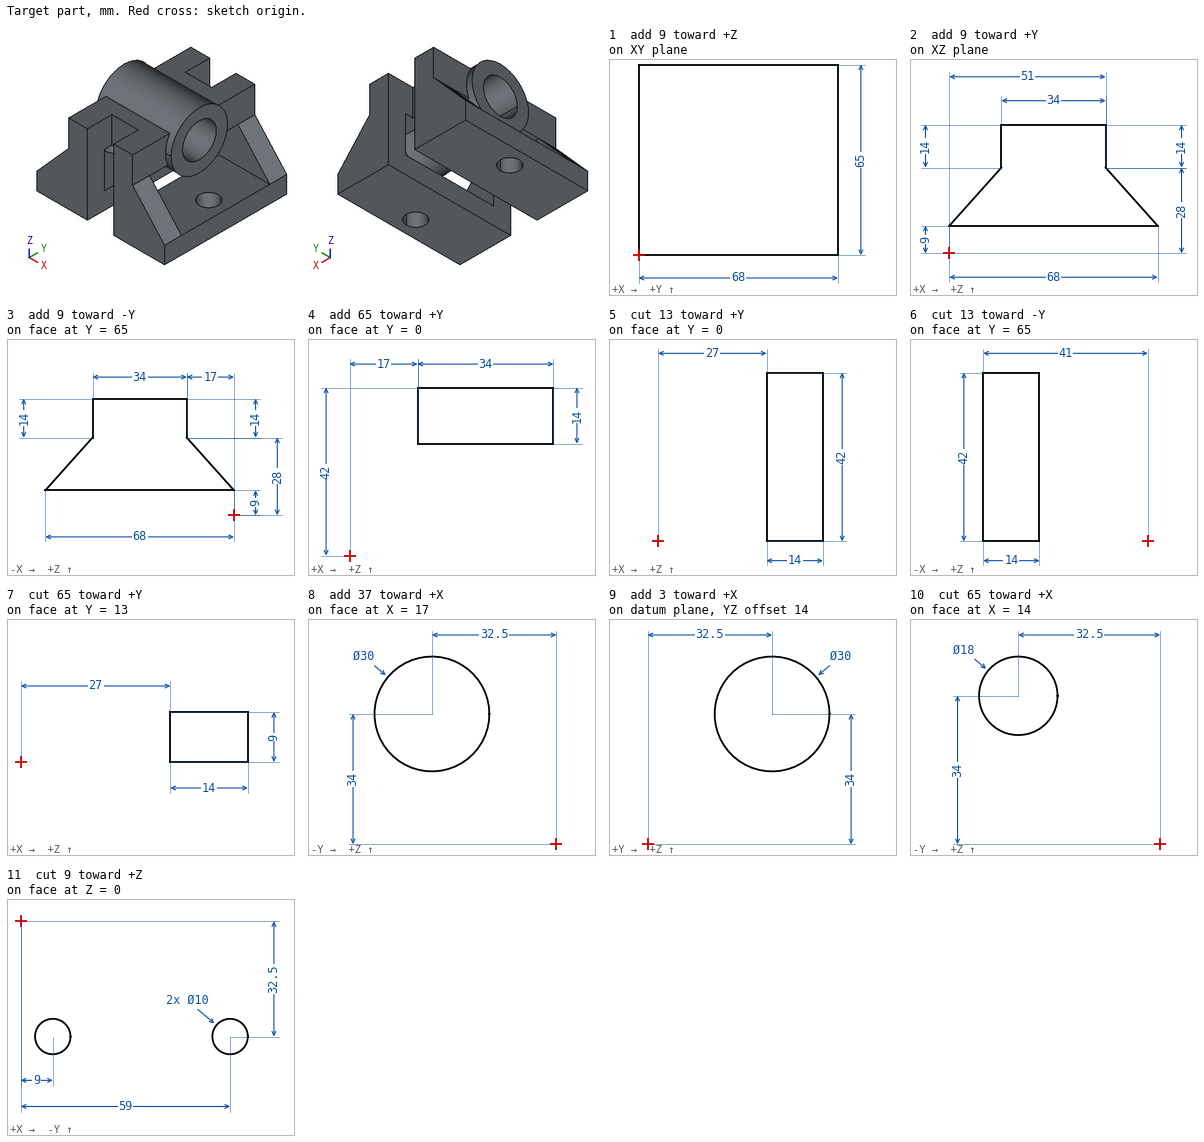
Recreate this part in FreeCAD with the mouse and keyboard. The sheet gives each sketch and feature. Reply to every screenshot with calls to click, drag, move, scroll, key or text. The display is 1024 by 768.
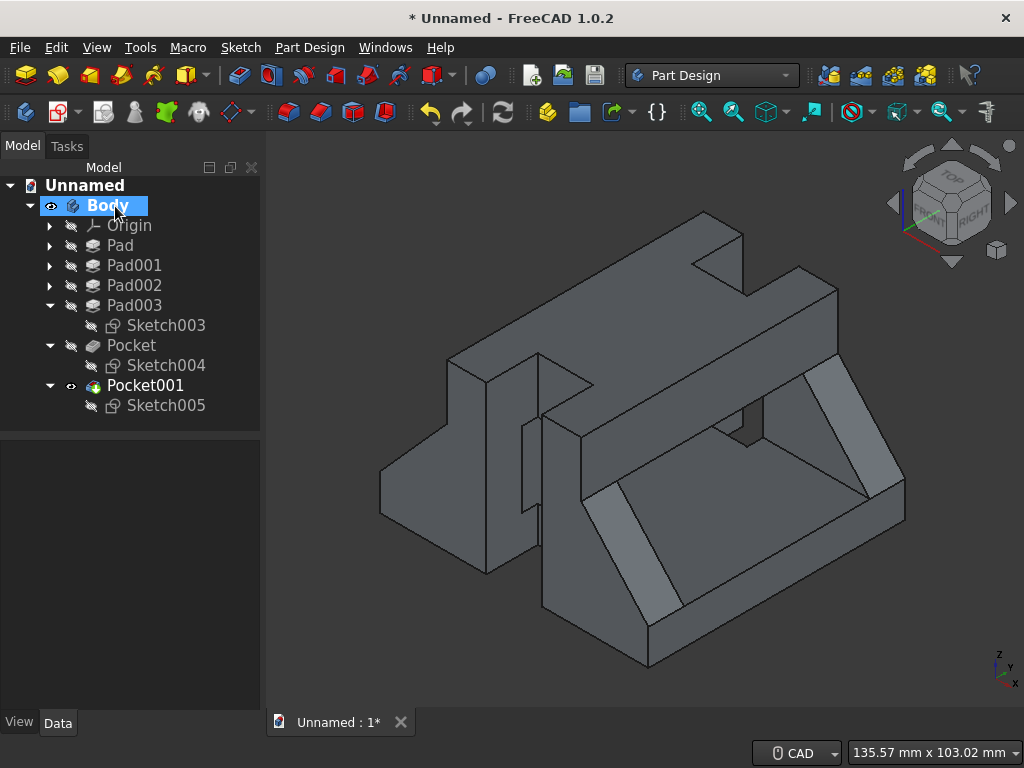
click(558, 386)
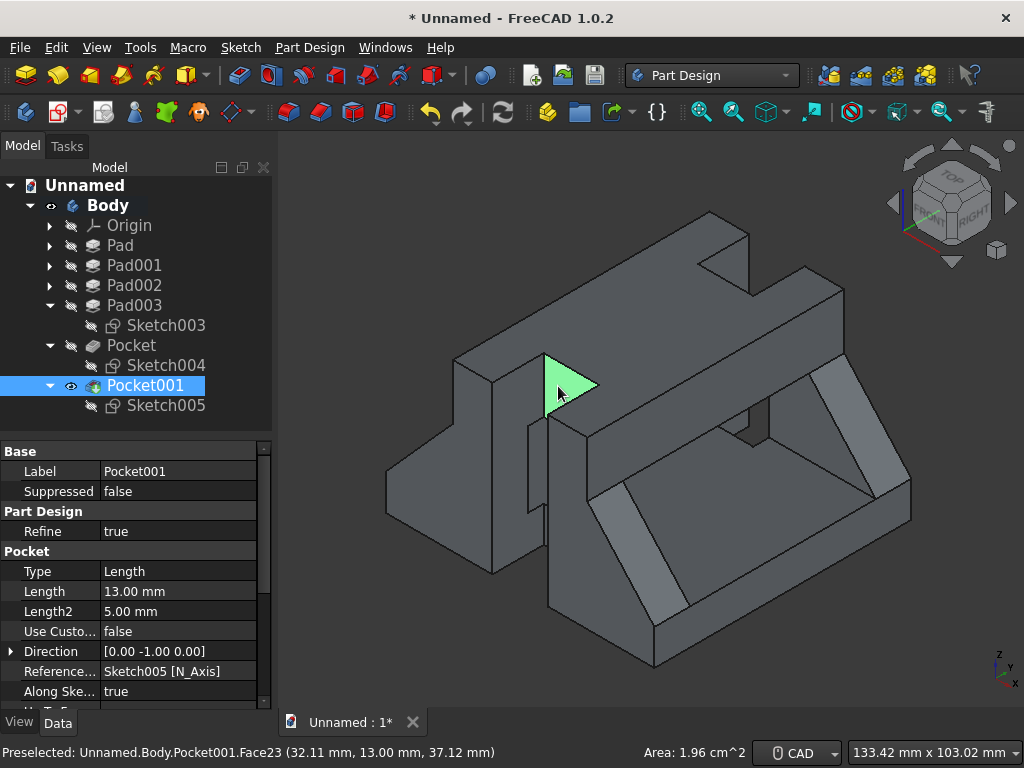
click(58, 112)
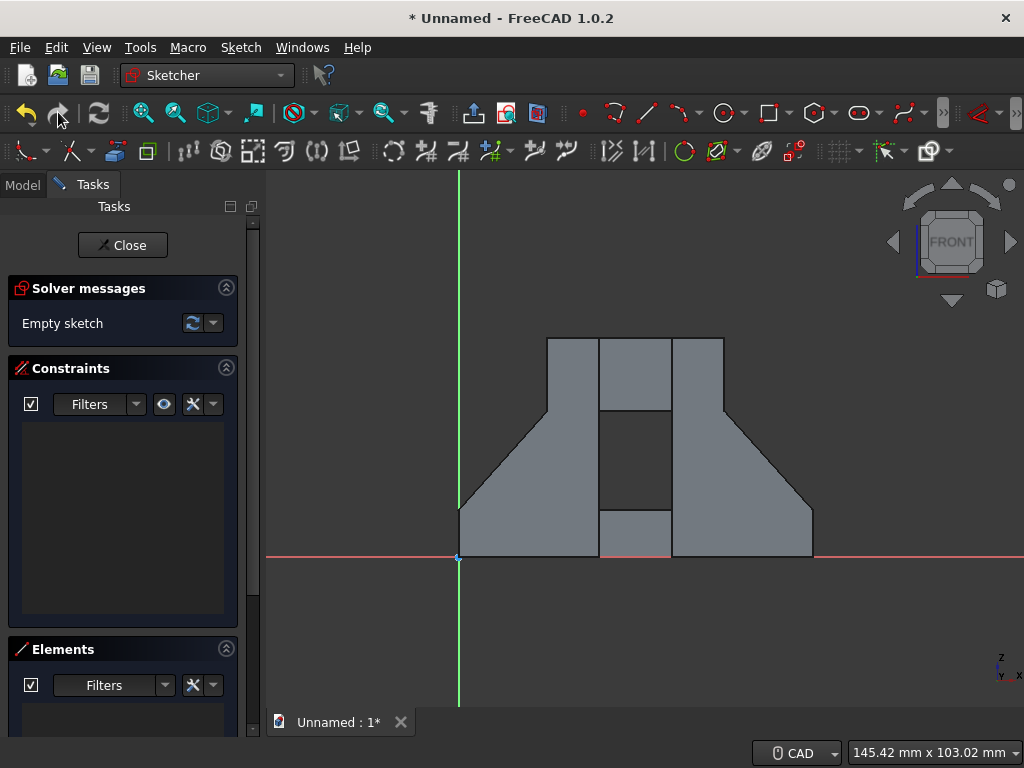
scroll(651, 558, up, 8)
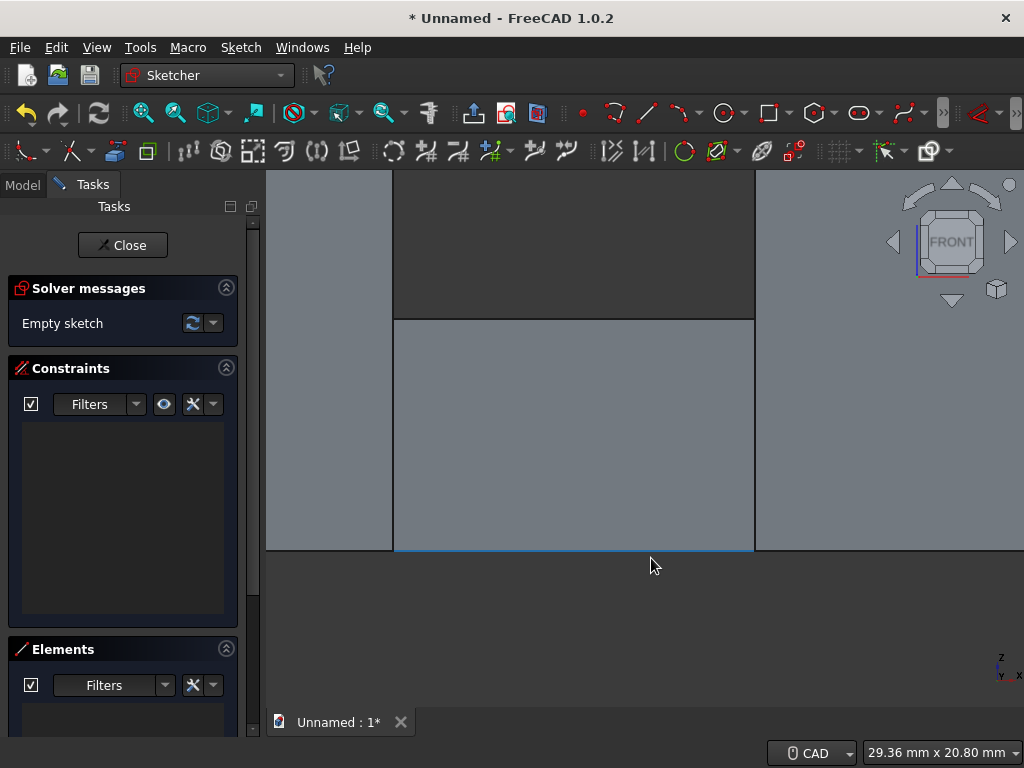
click(770, 114)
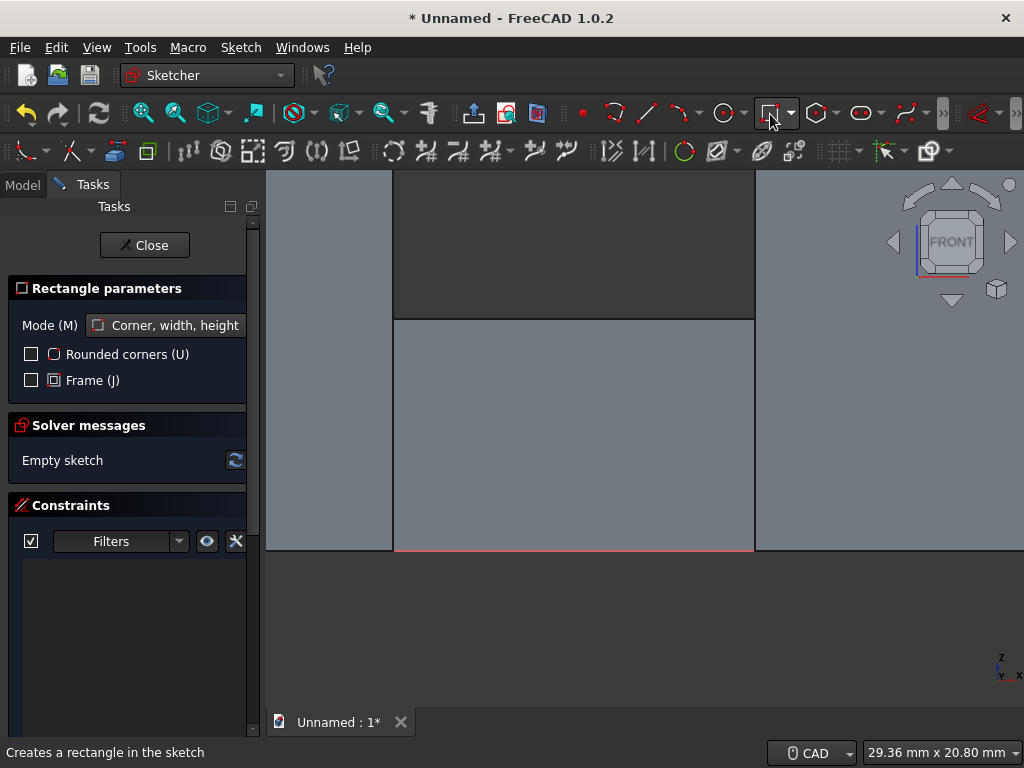
click(393, 319)
click(755, 551)
key(Escape)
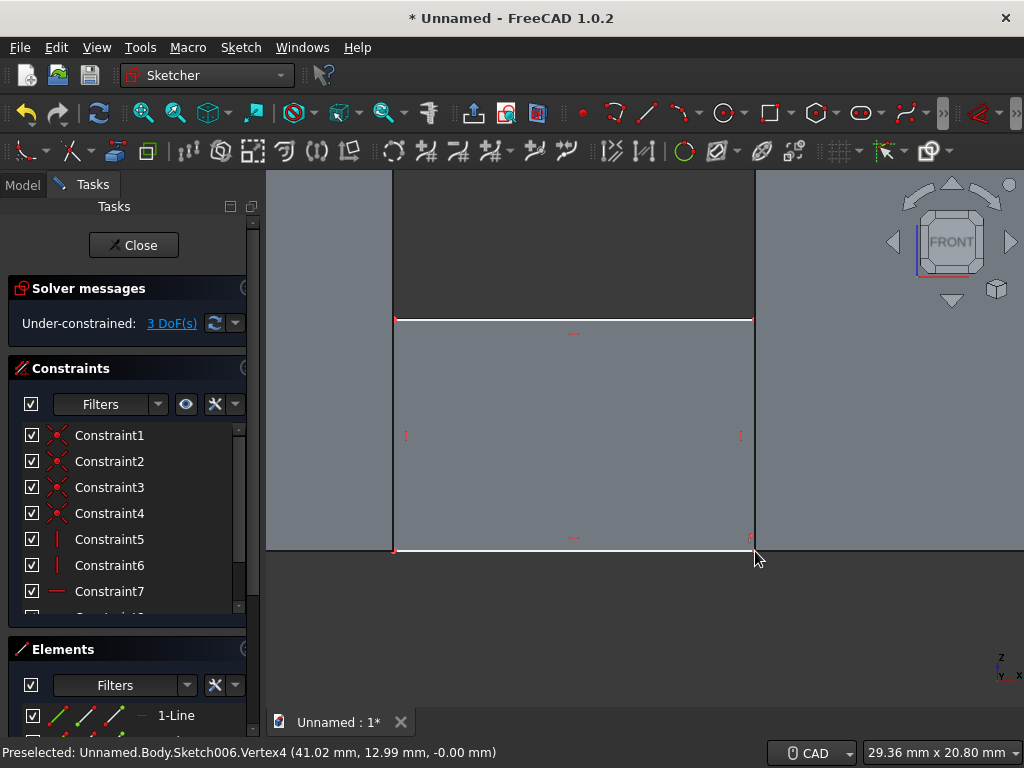
click(978, 114)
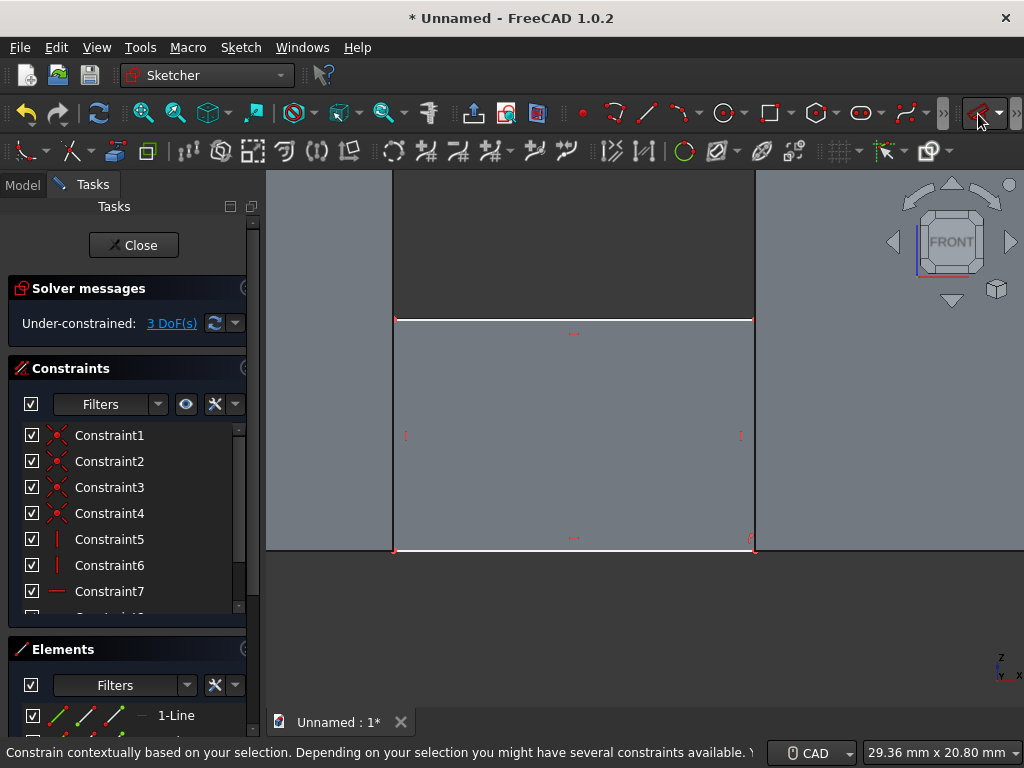
click(393, 389)
click(359, 435)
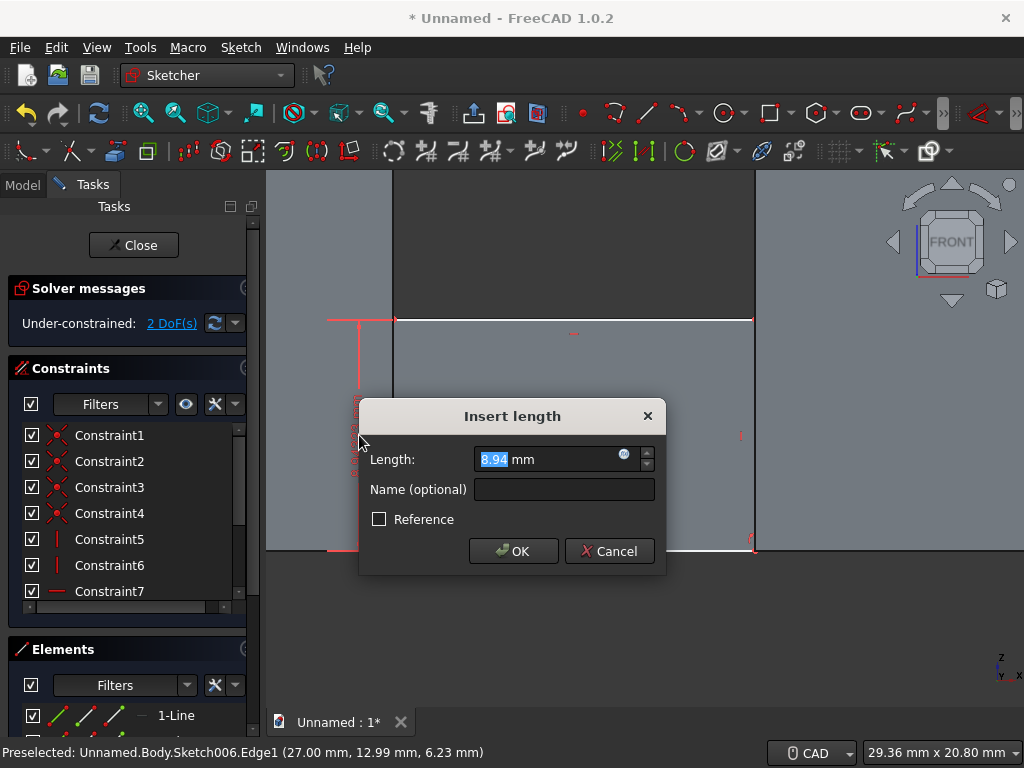
text(9)
key(Return)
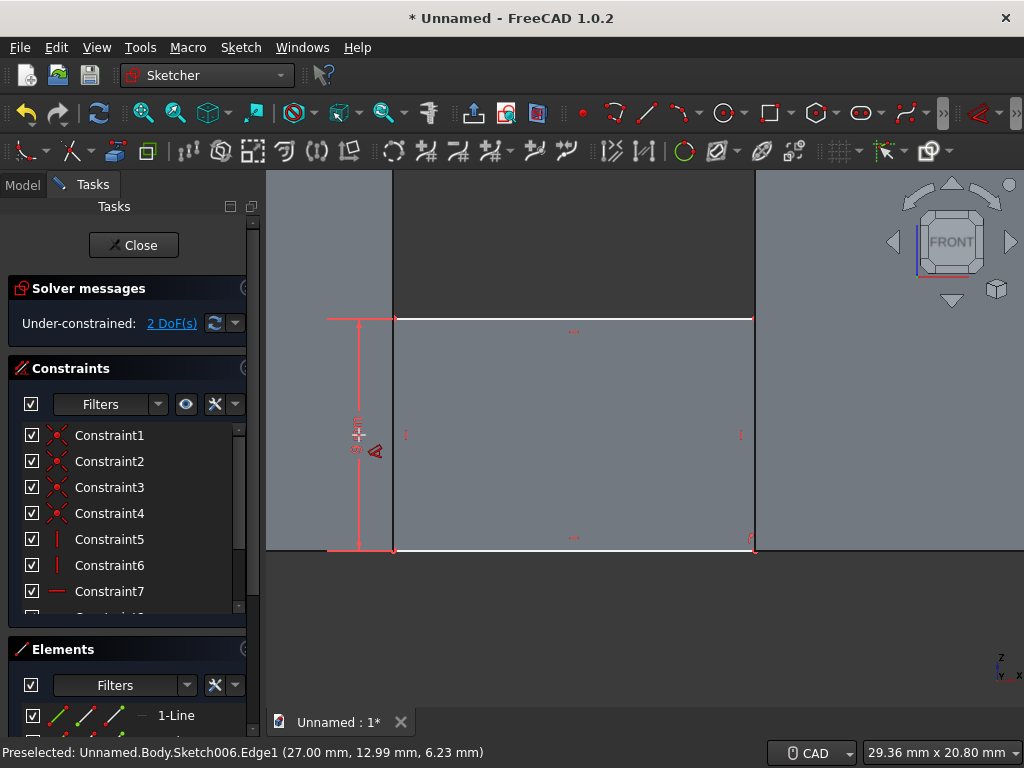
click(502, 551)
click(574, 585)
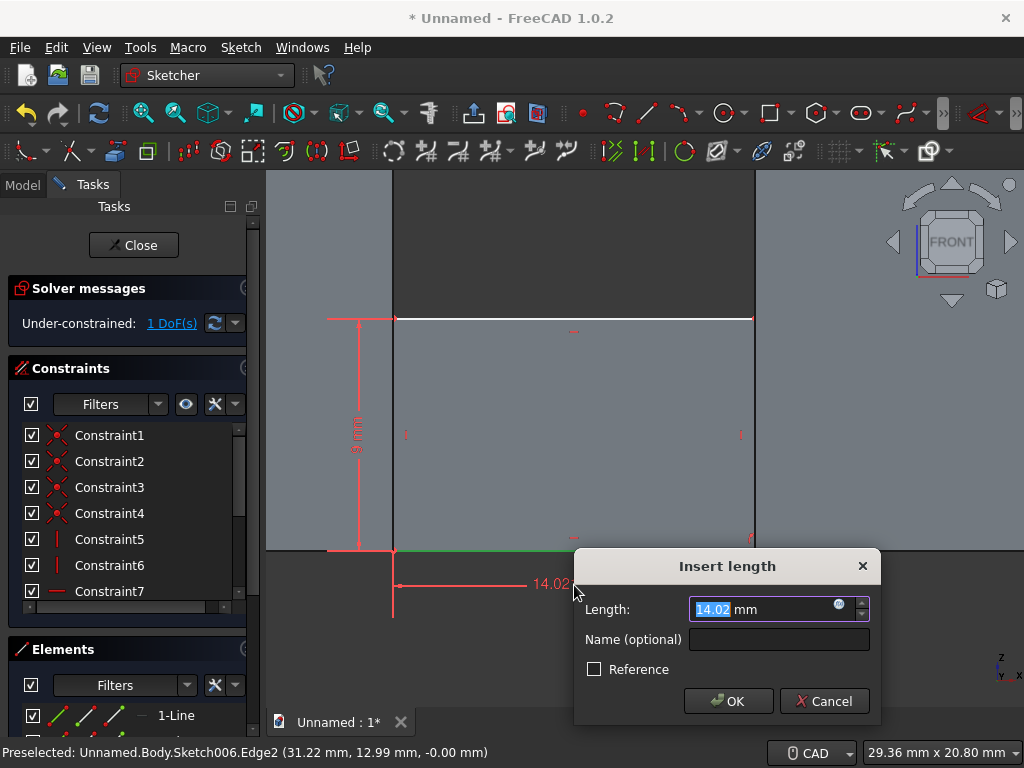
text(14)
key(Return)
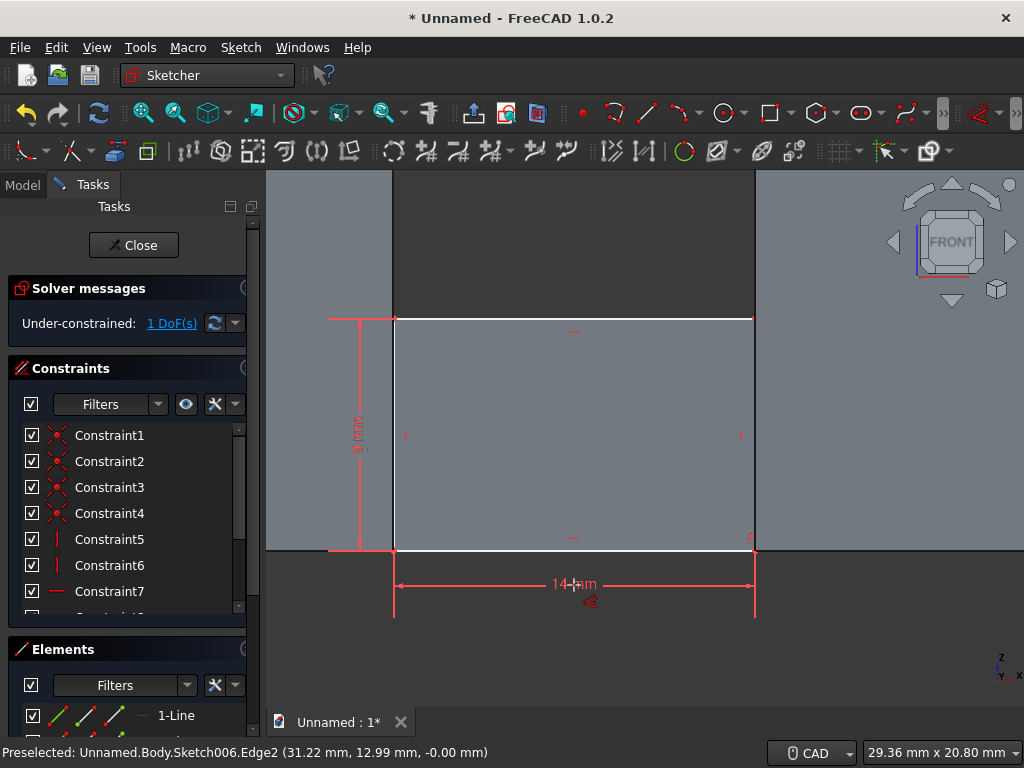
click(394, 319)
click(344, 585)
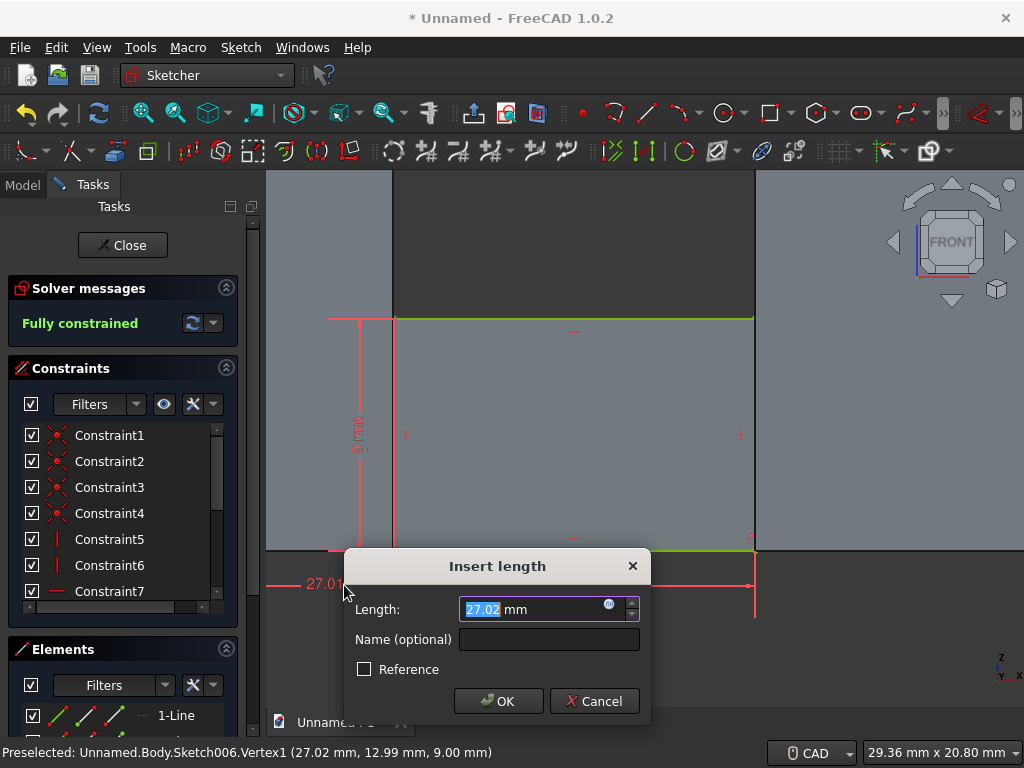
text(27)
key(Return)
key(Escape)